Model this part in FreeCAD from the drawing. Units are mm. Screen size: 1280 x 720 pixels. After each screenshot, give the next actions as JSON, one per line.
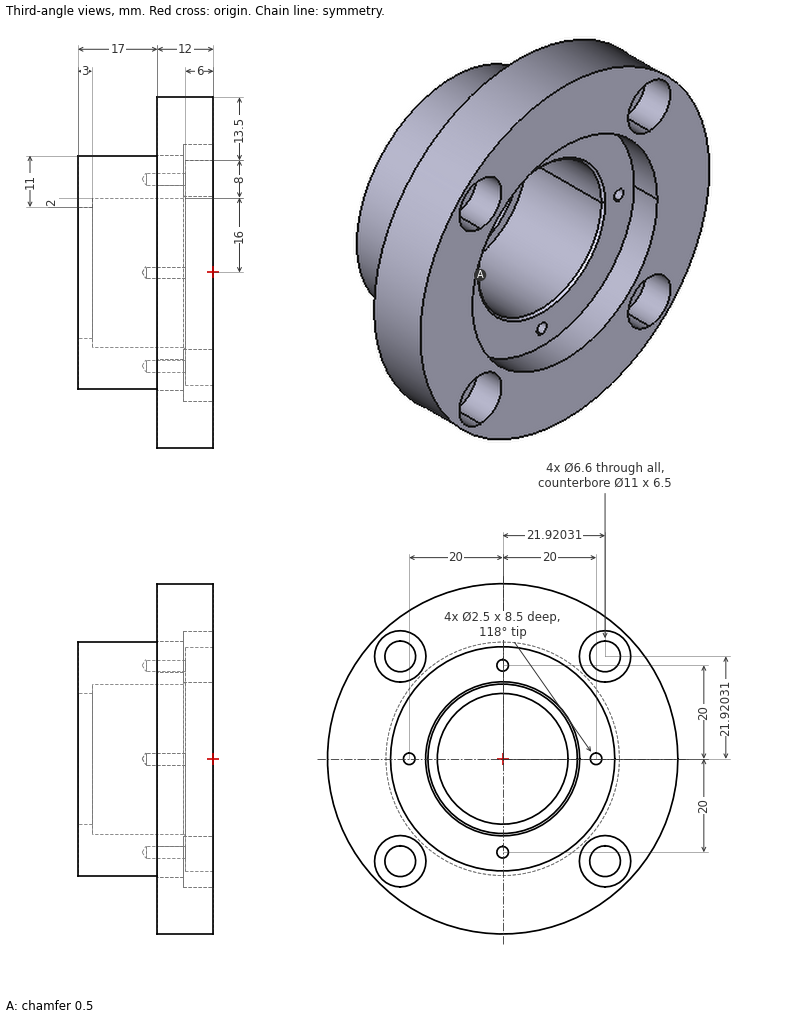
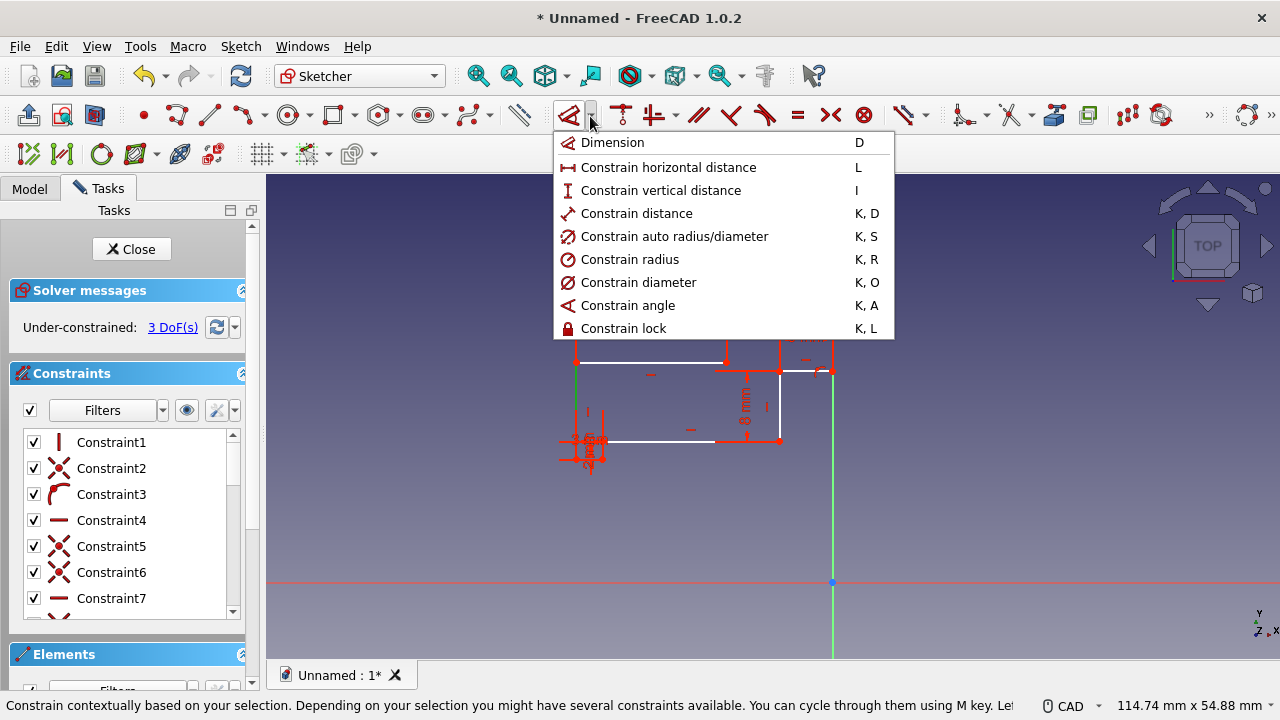
{"action": "left_click", "coordinate": [724, 190]}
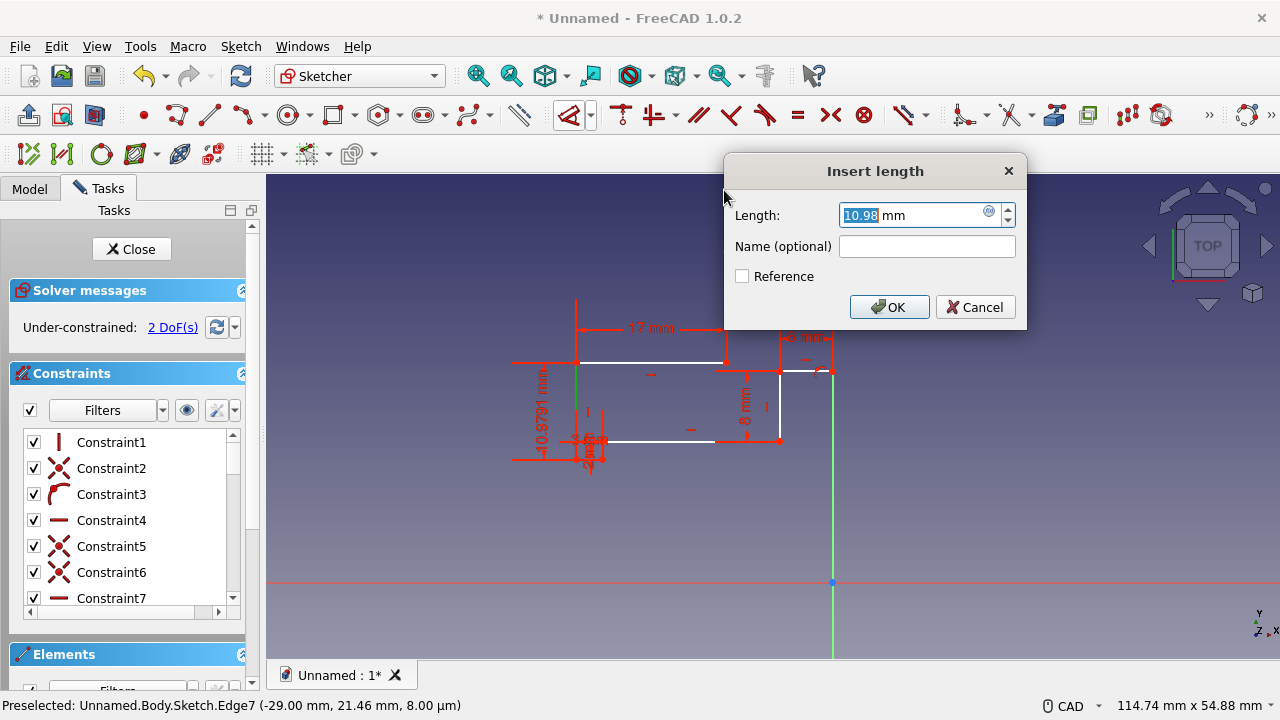
{"action": "type", "text": "11"}
{"action": "key", "text": "Return"}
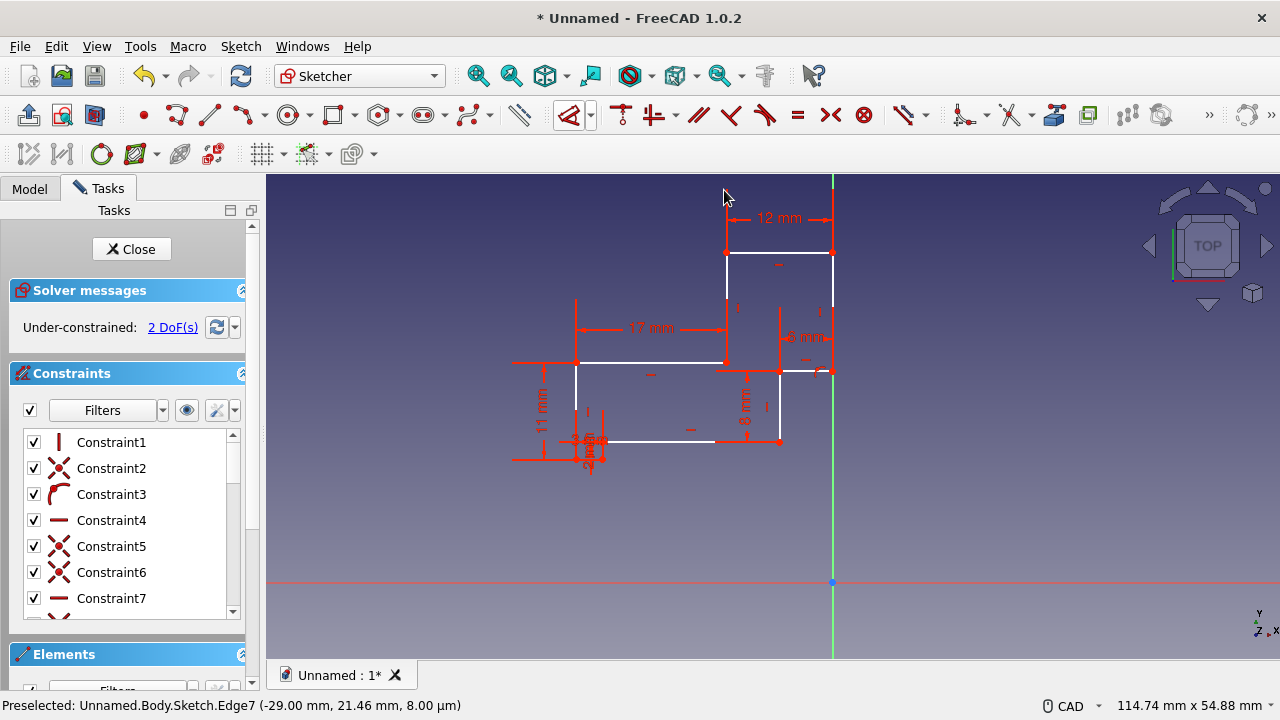
{"action": "left_click", "coordinate": [780, 442]}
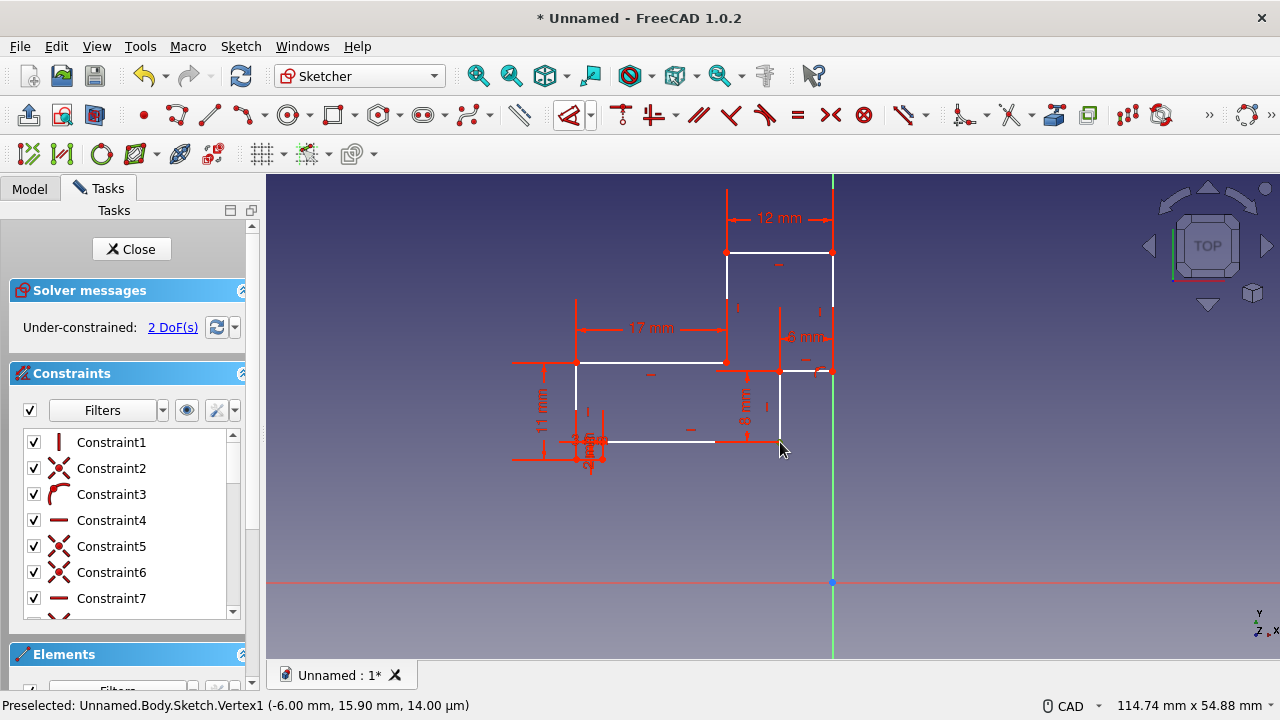
{"action": "key", "text": "i"}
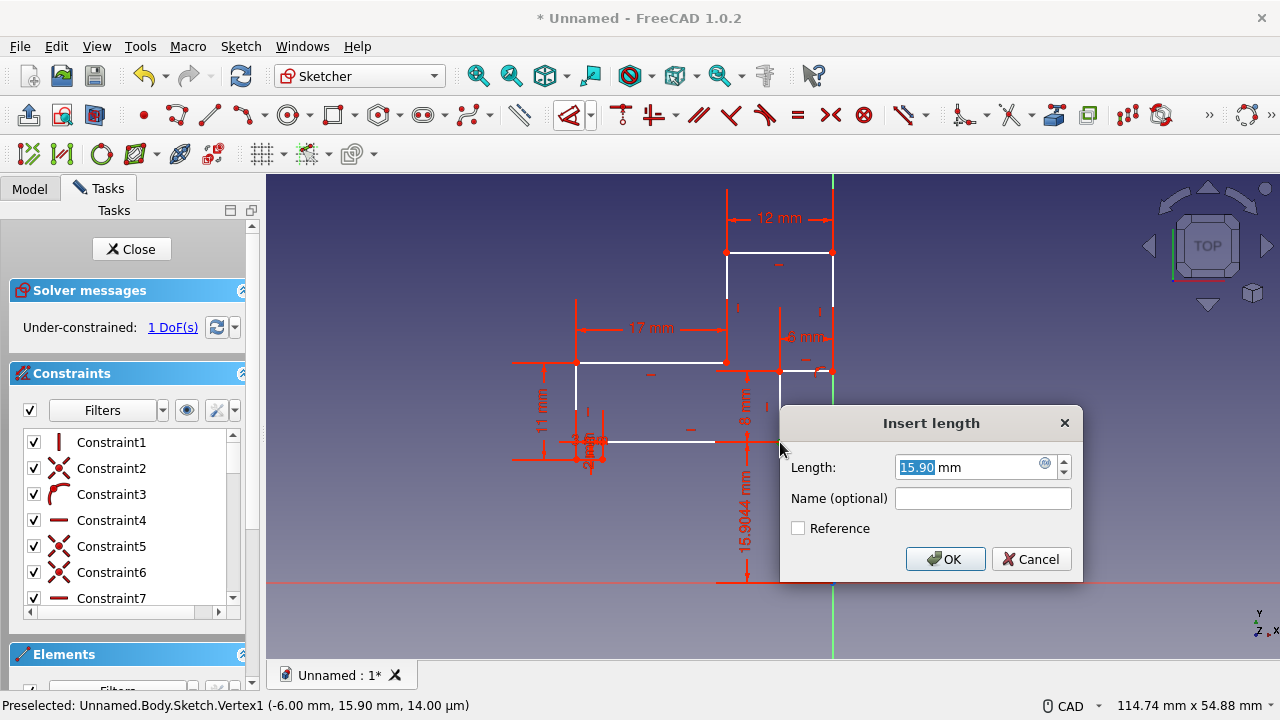
{"action": "type", "text": "16"}
{"action": "key", "text": "Return"}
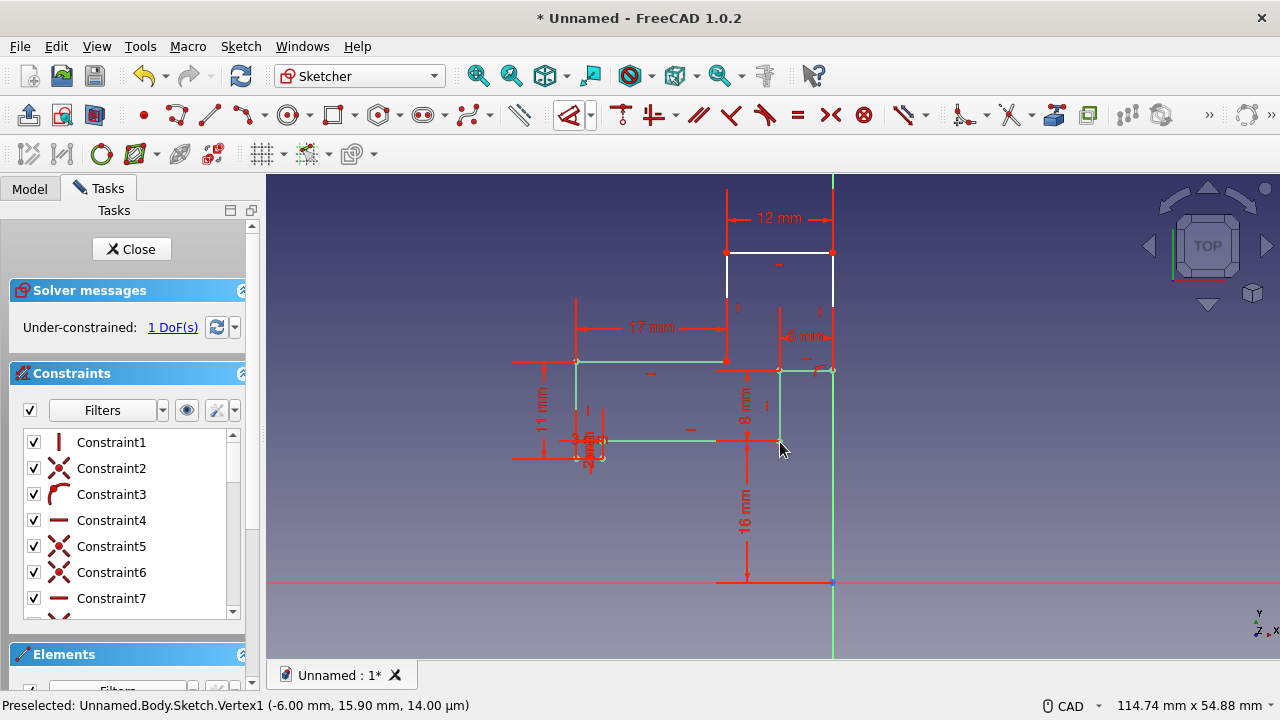
{"action": "left_click", "coordinate": [833, 335]}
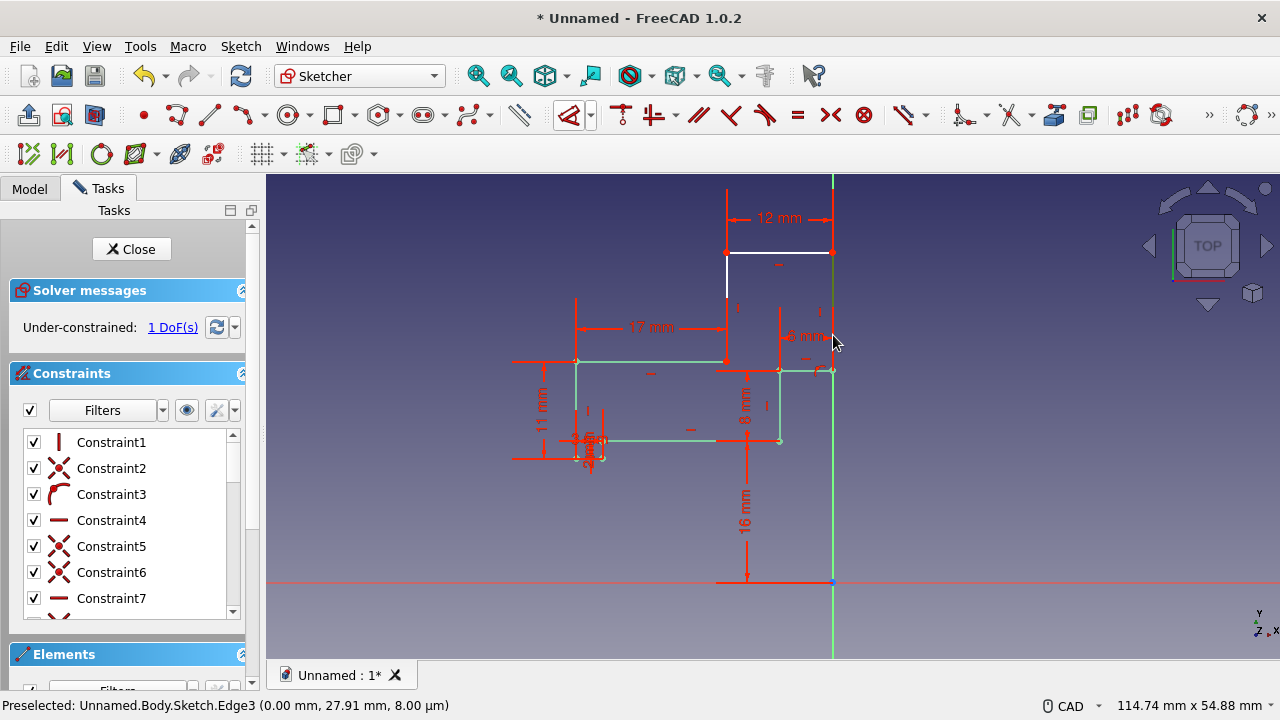
{"action": "key", "text": "i"}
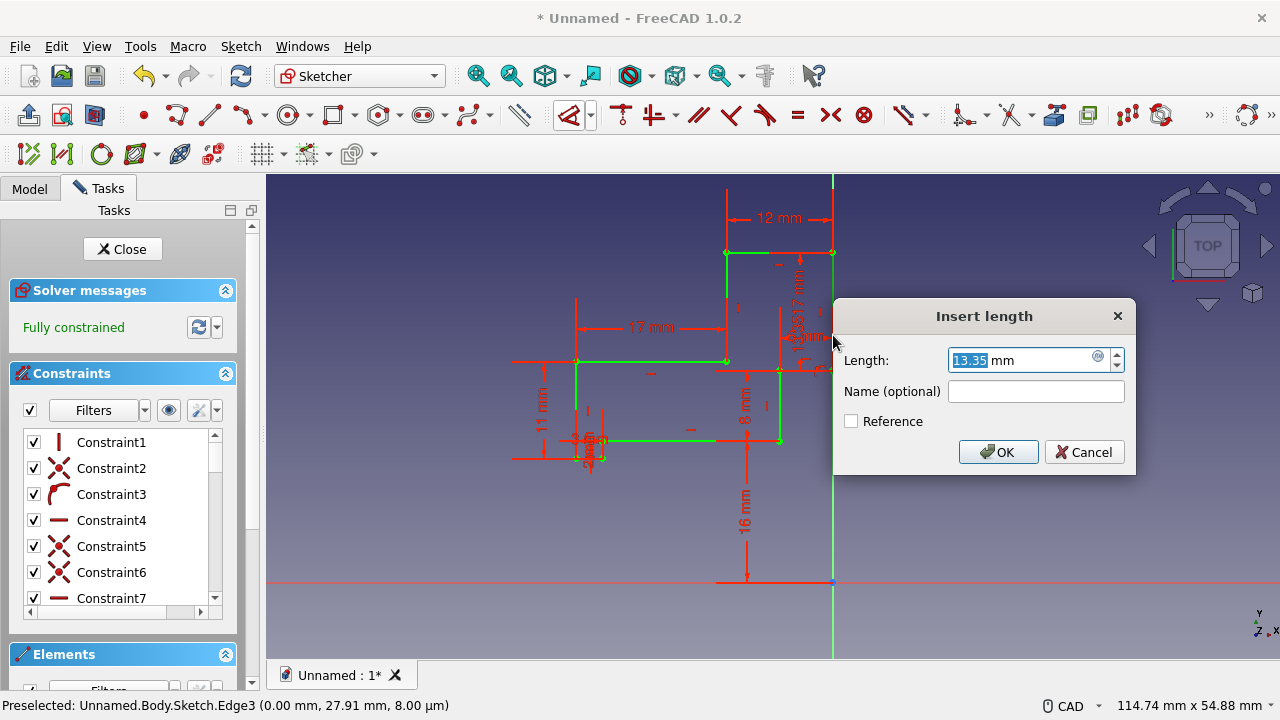
{"action": "type", "text": "13.5"}
{"action": "key", "text": "Return"}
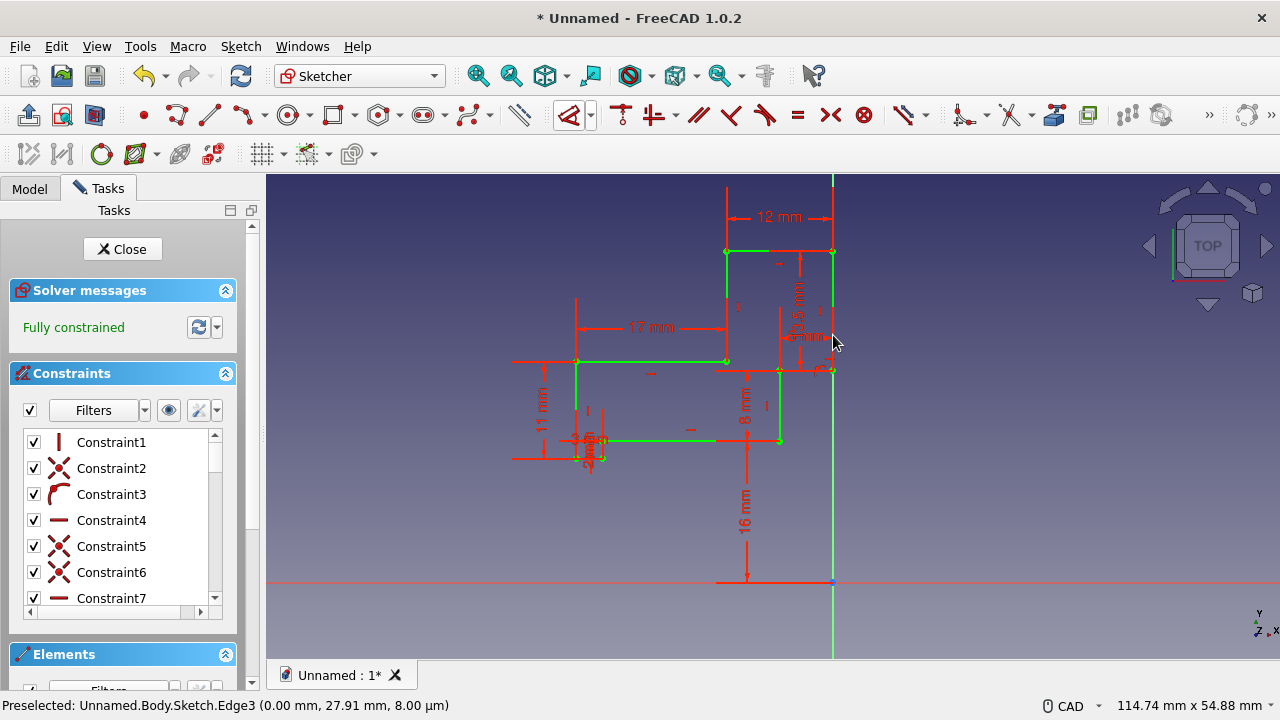
{"action": "left_click", "coordinate": [123, 249]}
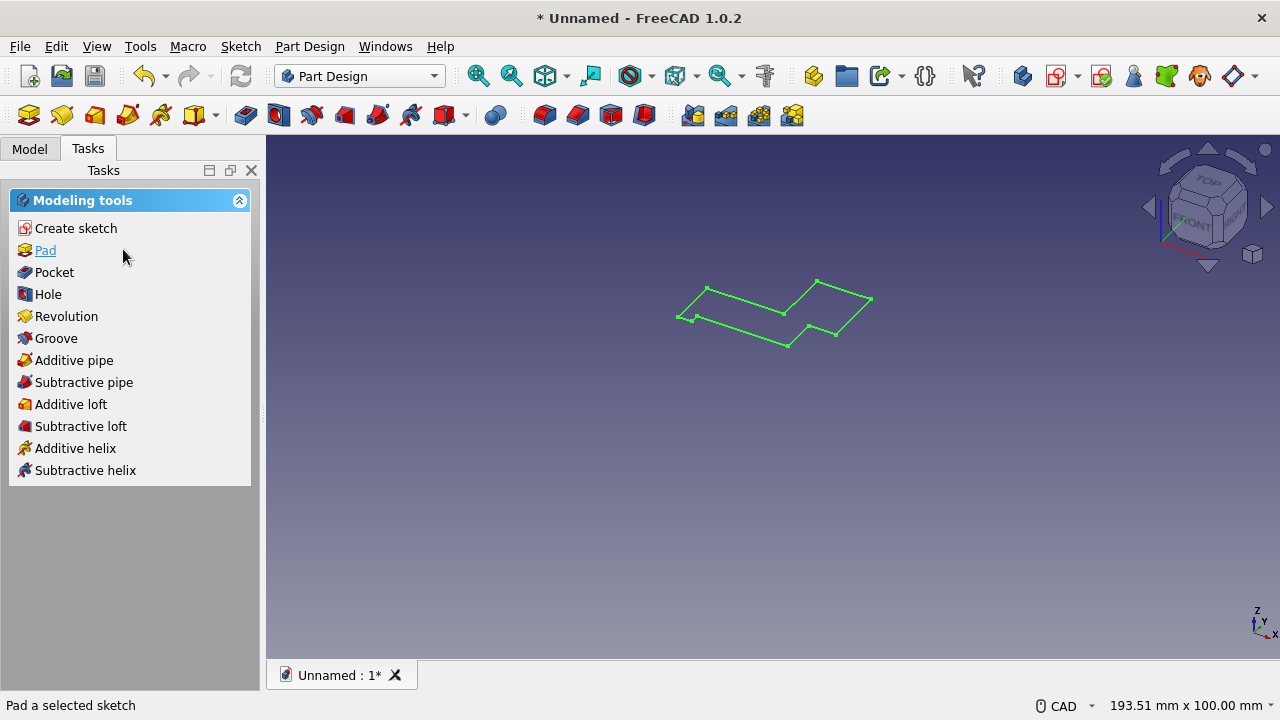
{"action": "left_click", "coordinate": [62, 116]}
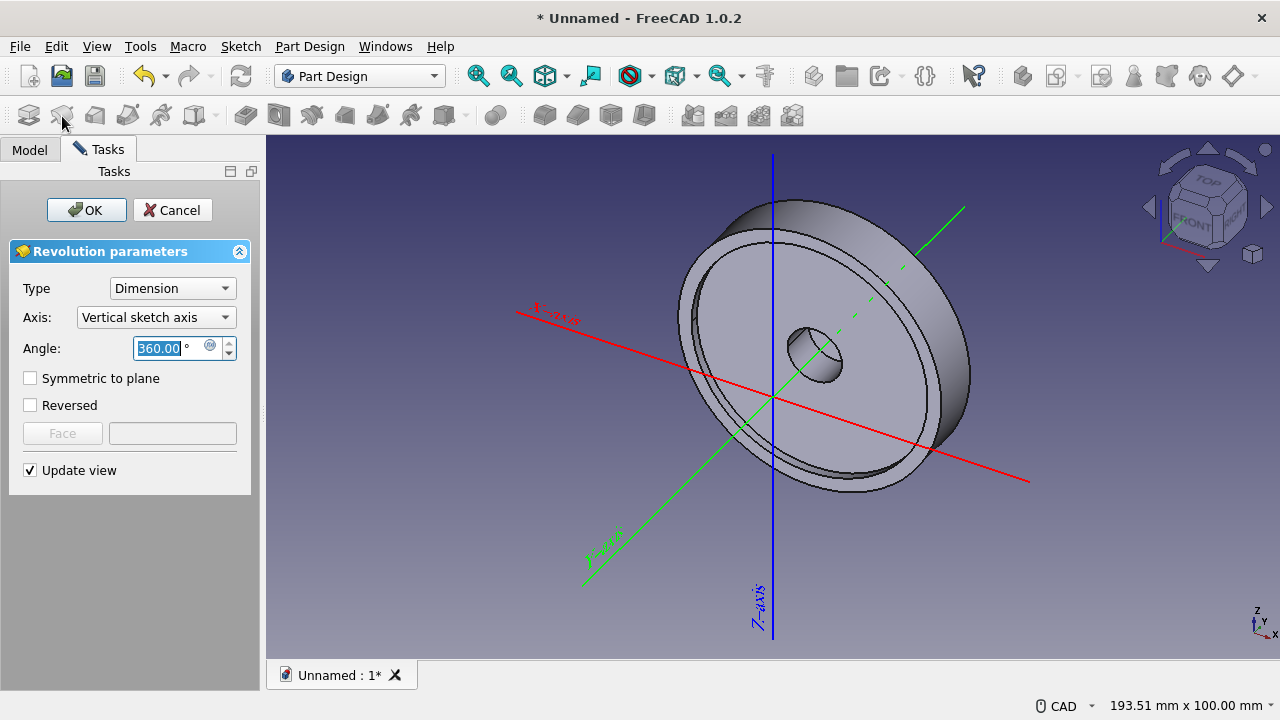
{"action": "left_click", "coordinate": [157, 318]}